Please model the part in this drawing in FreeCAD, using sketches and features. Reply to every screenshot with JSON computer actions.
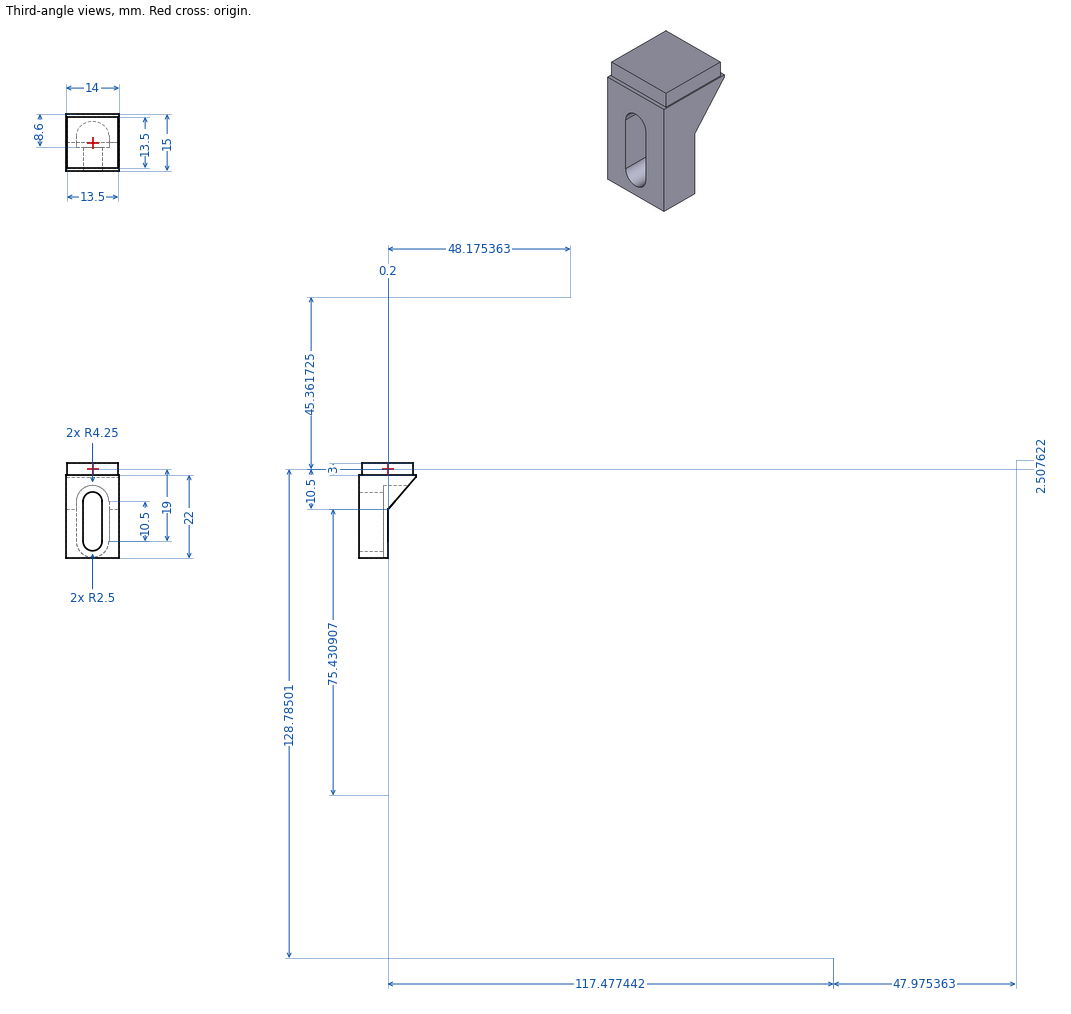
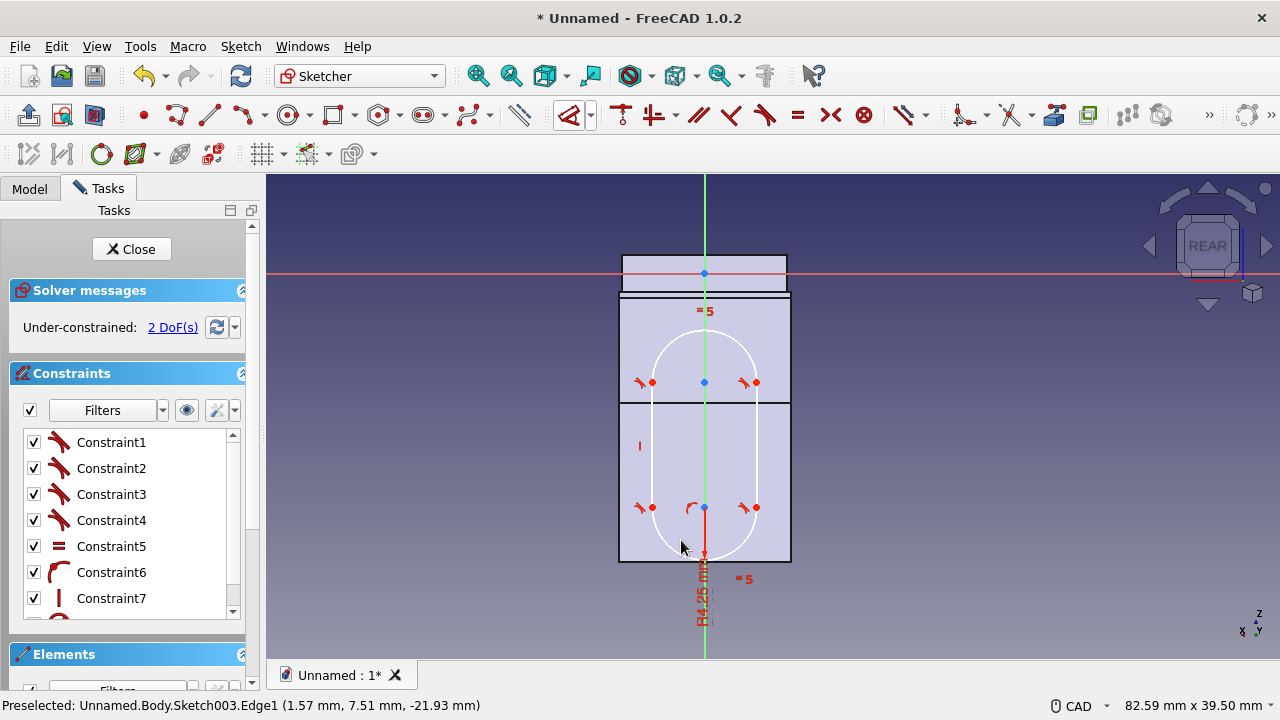
{"action": "left_click", "coordinate": [652, 508]}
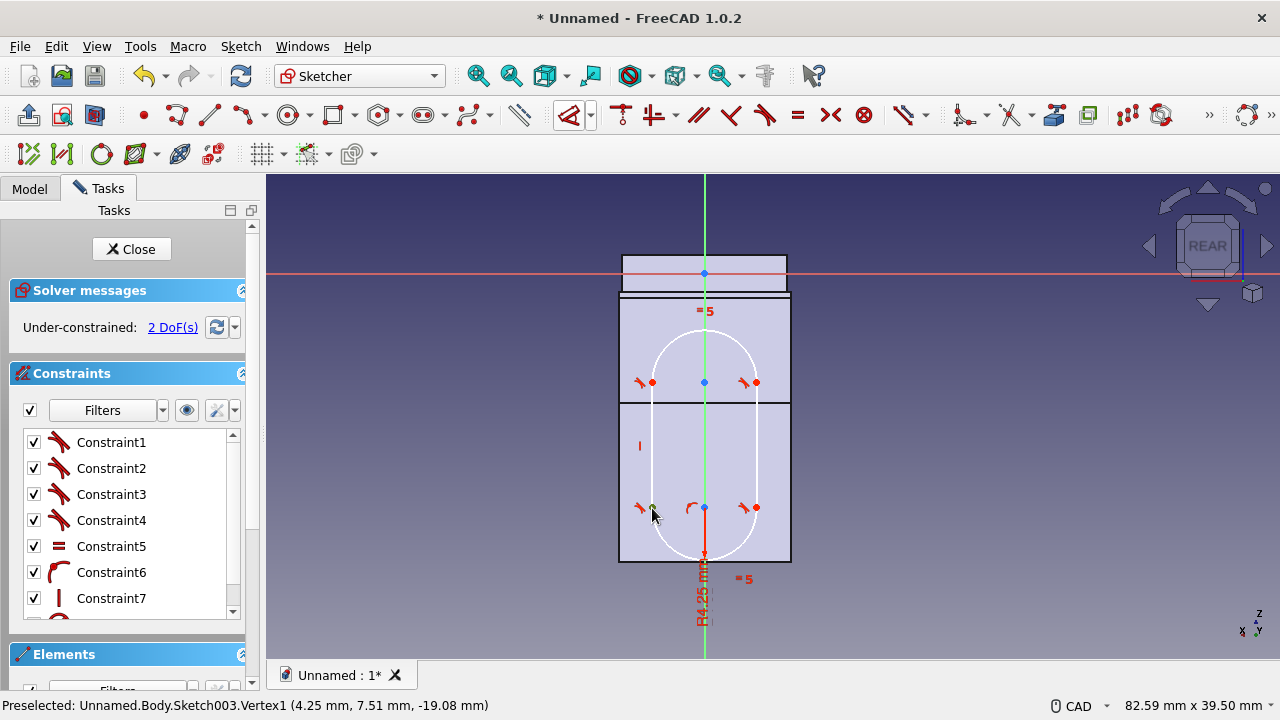
{"action": "left_click", "coordinate": [590, 116]}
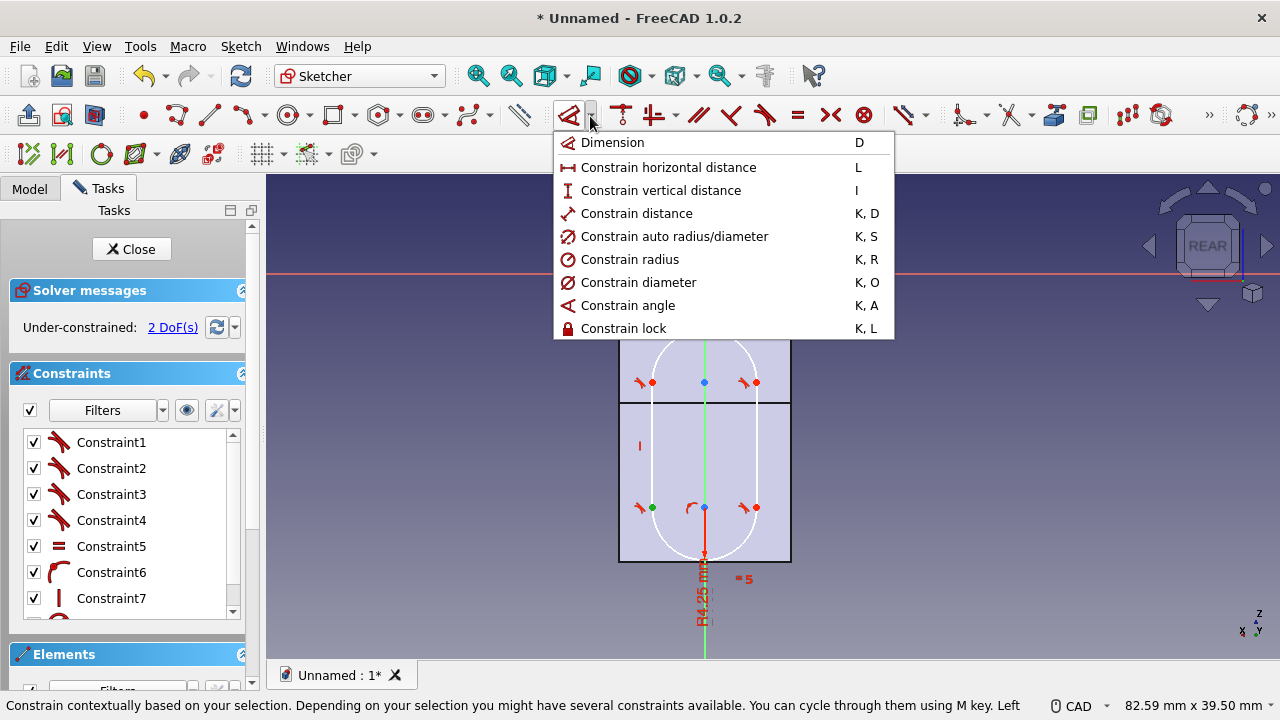
{"action": "left_click", "coordinate": [724, 190]}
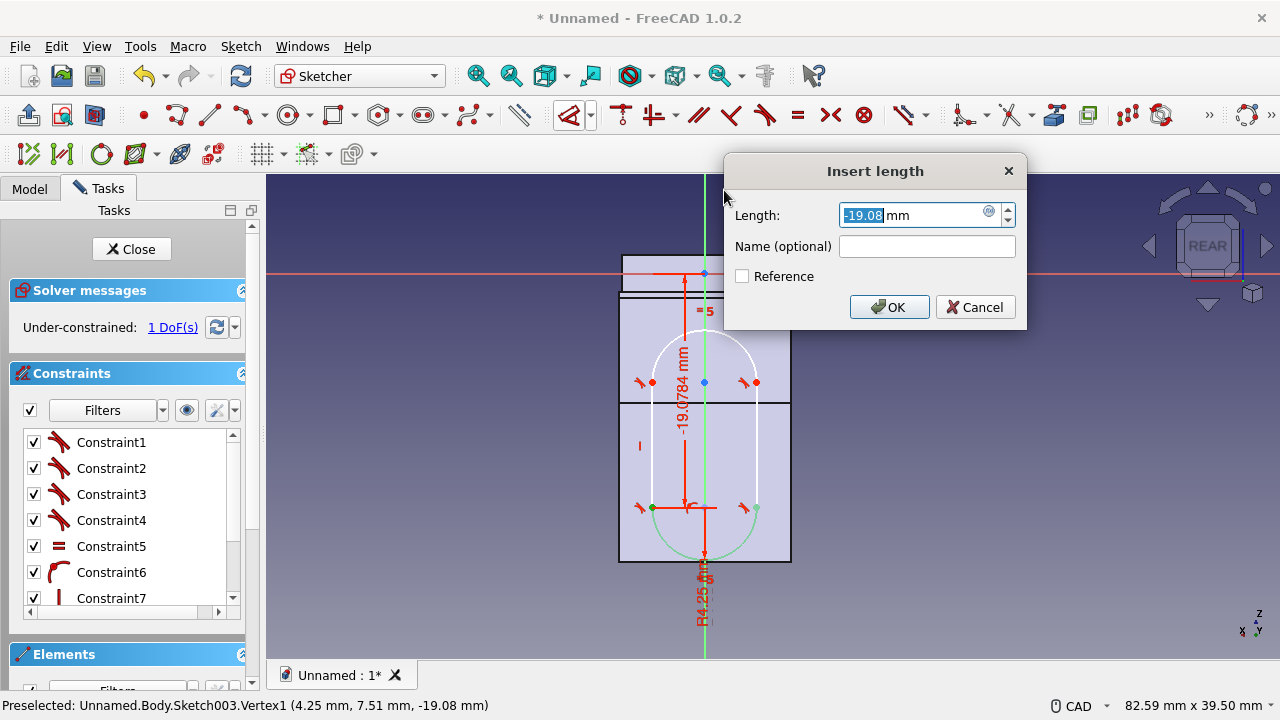
{"action": "type", "text": "-19"}
{"action": "key", "text": "Return"}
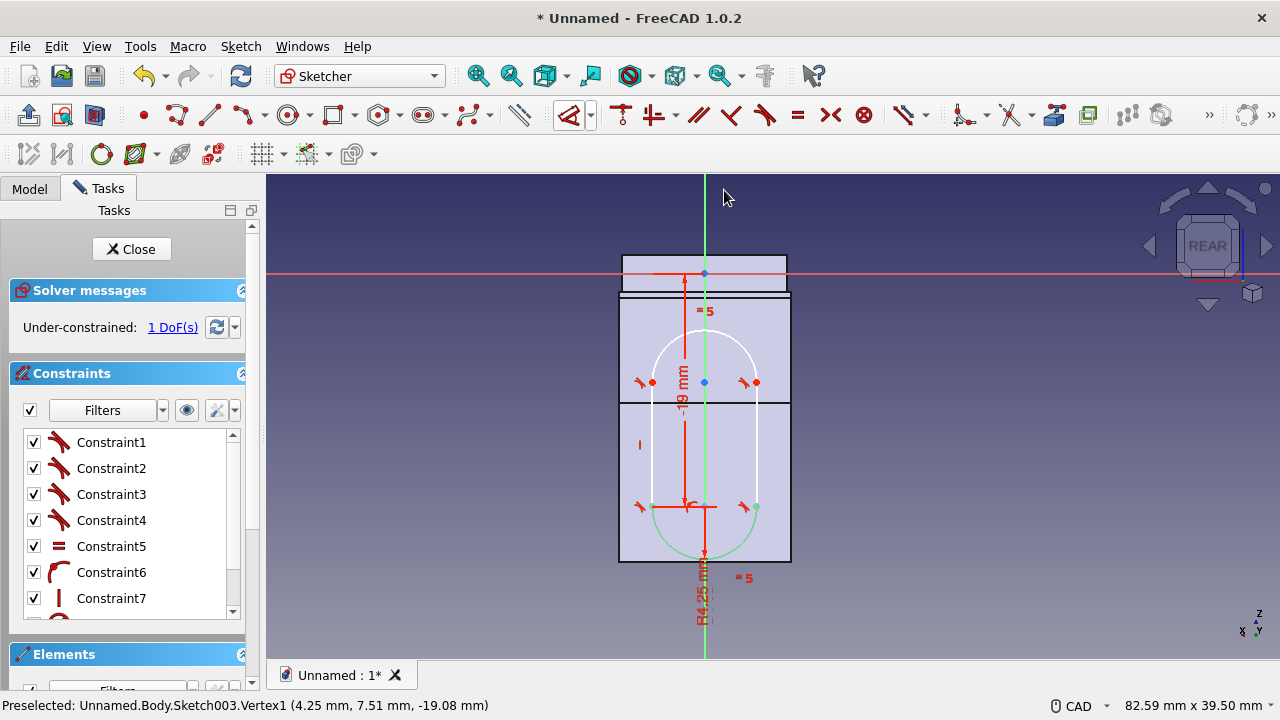
{"action": "left_click", "coordinate": [652, 470]}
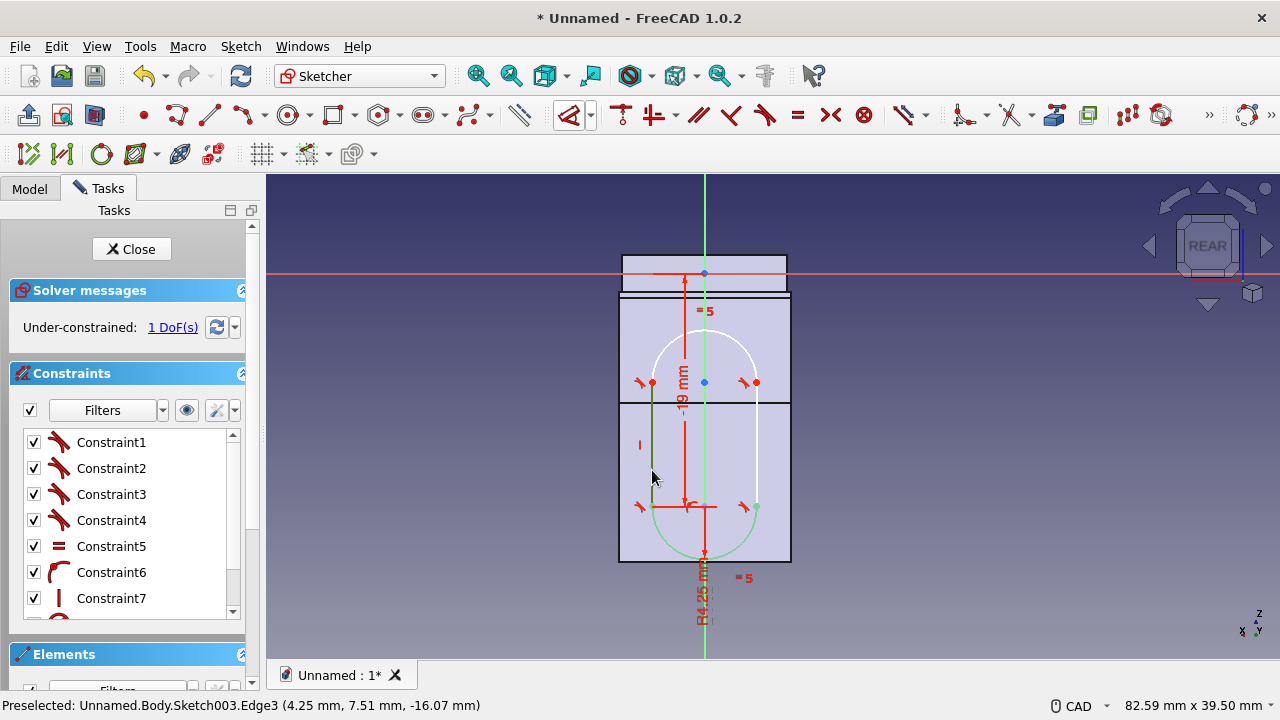
{"action": "key", "text": "i"}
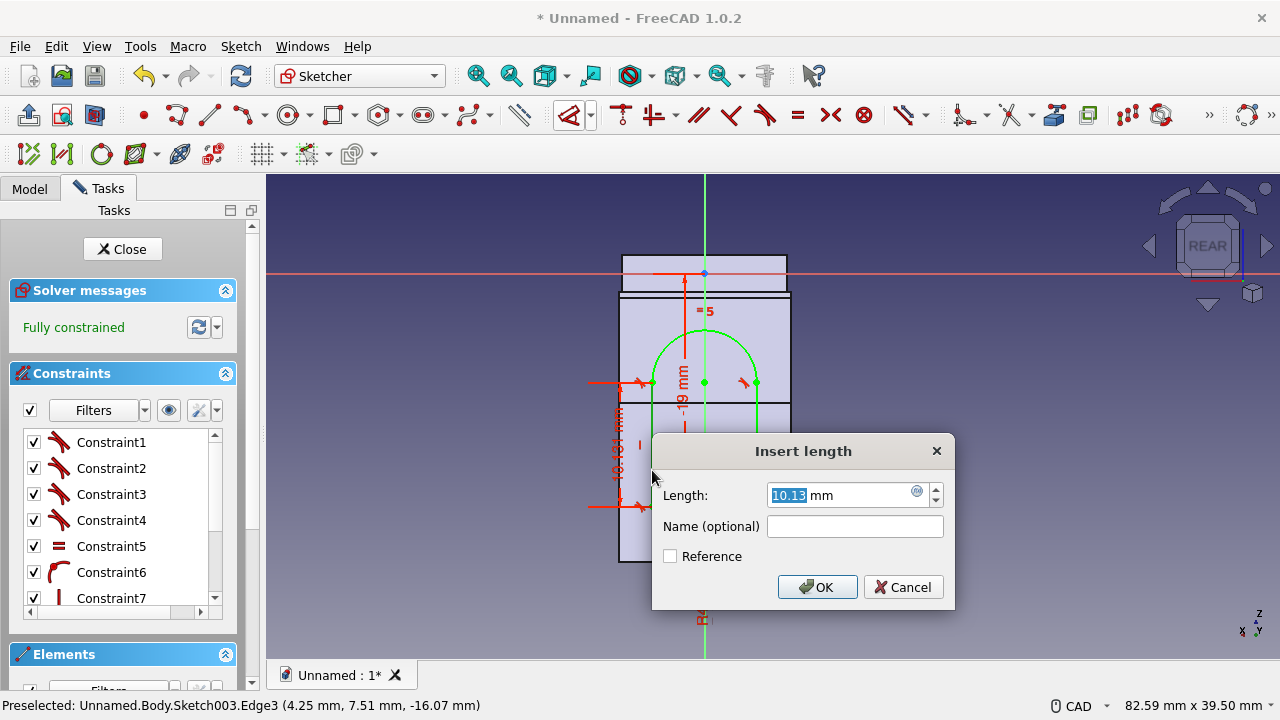
{"action": "type", "text": "10.5"}
{"action": "key", "text": "Return"}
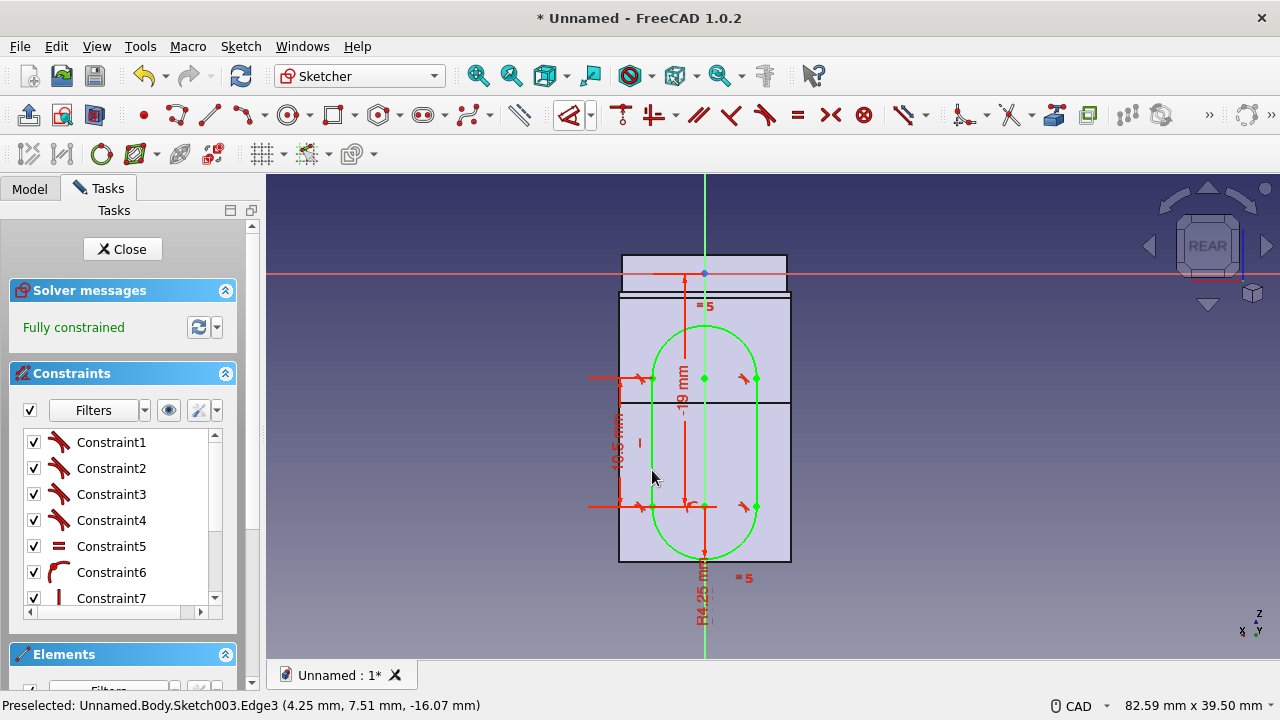
{"action": "left_click", "coordinate": [123, 249]}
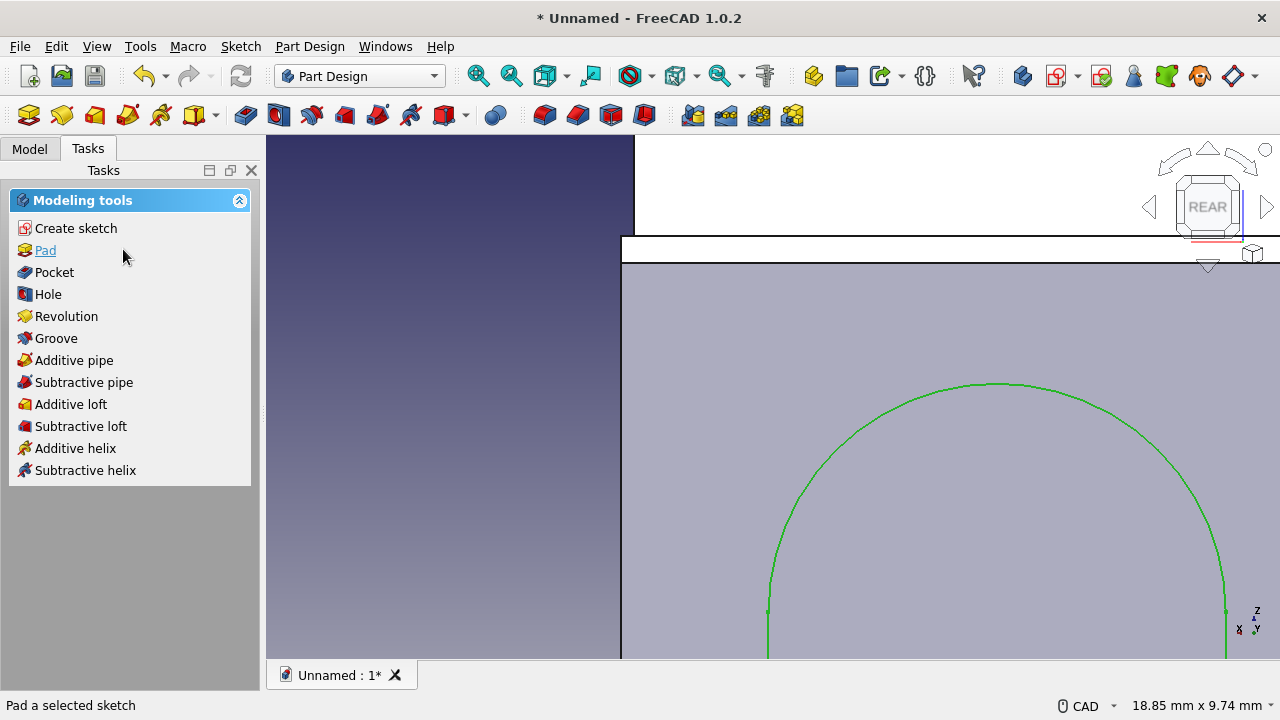
{"action": "left_click", "coordinate": [246, 116]}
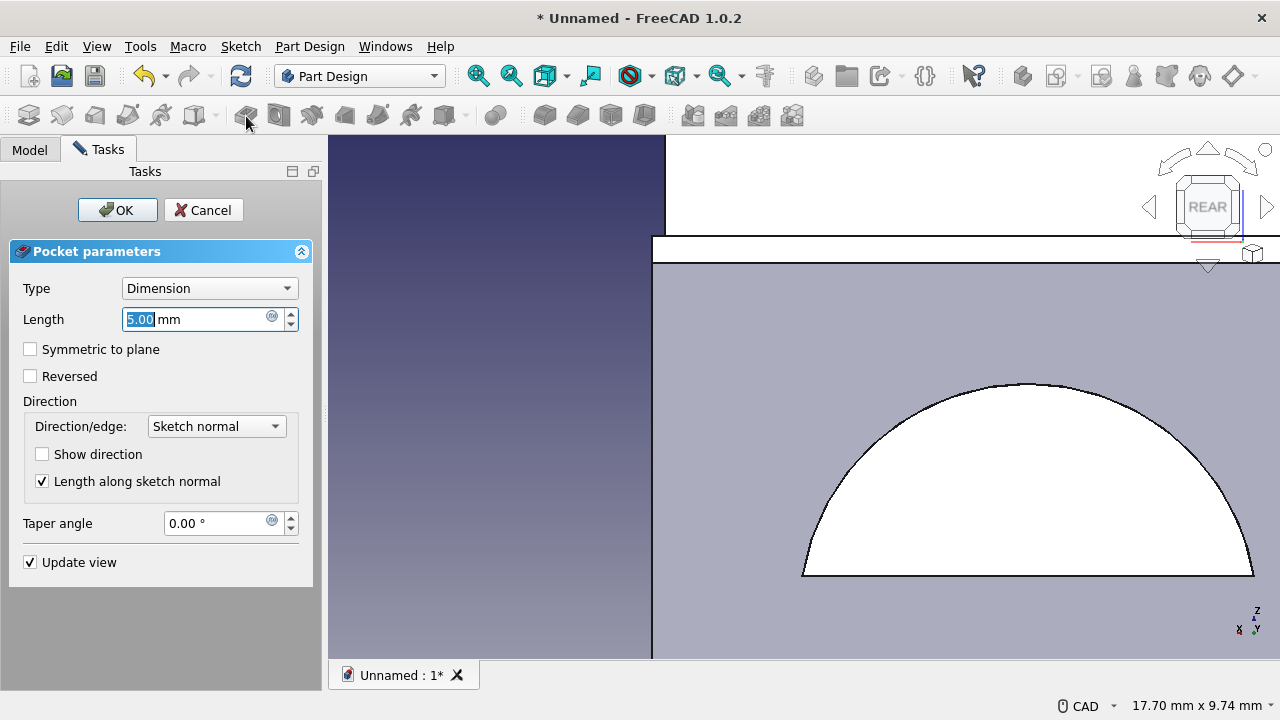
{"action": "type", "text": "8.6"}
{"action": "key", "text": "Tab"}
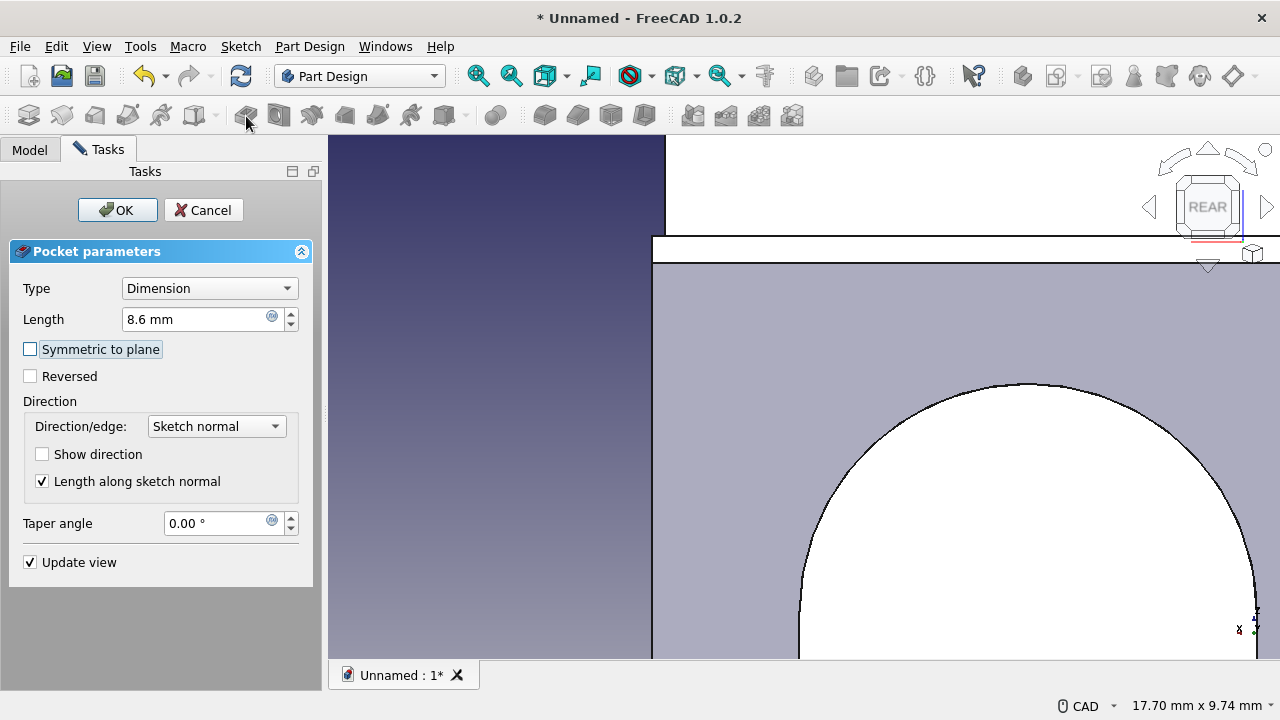
{"action": "left_click", "coordinate": [118, 210]}